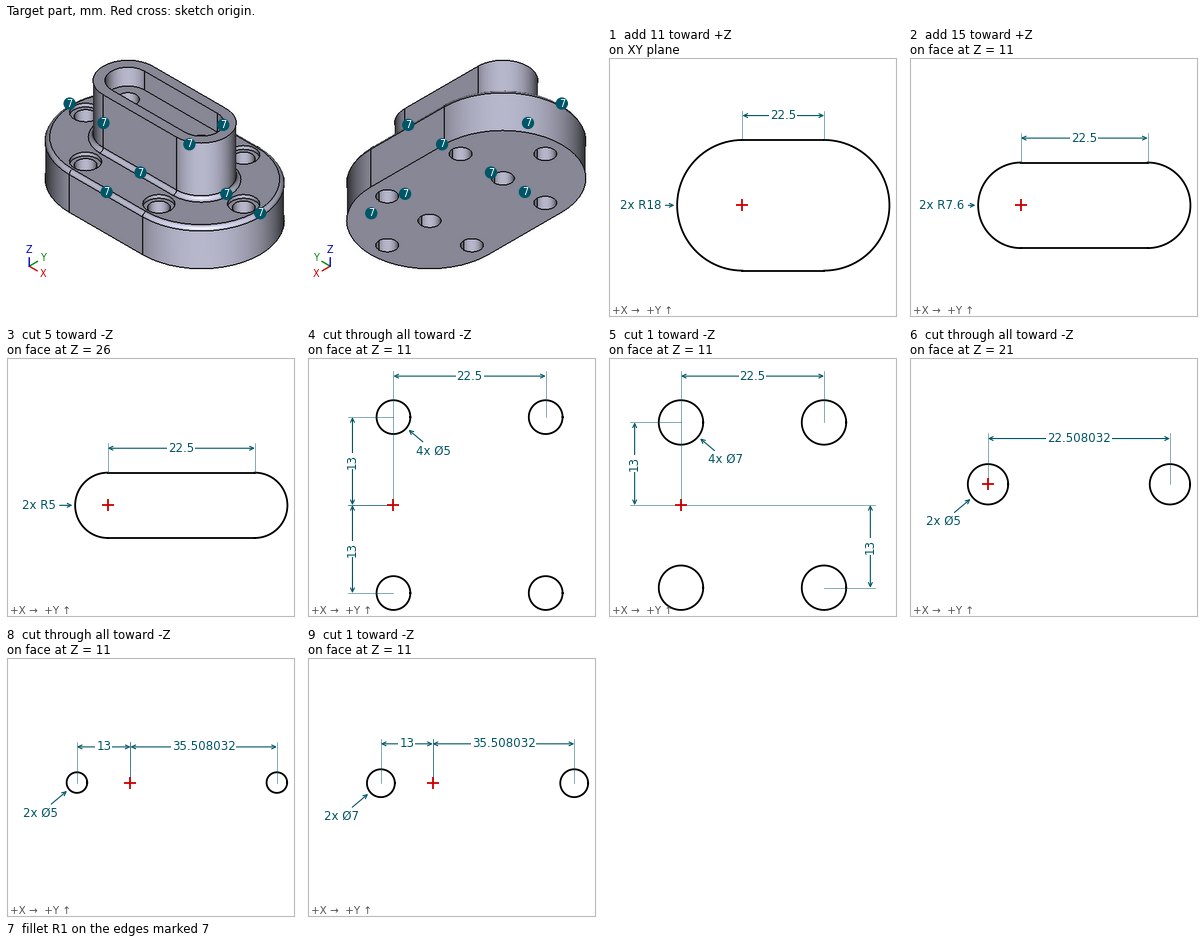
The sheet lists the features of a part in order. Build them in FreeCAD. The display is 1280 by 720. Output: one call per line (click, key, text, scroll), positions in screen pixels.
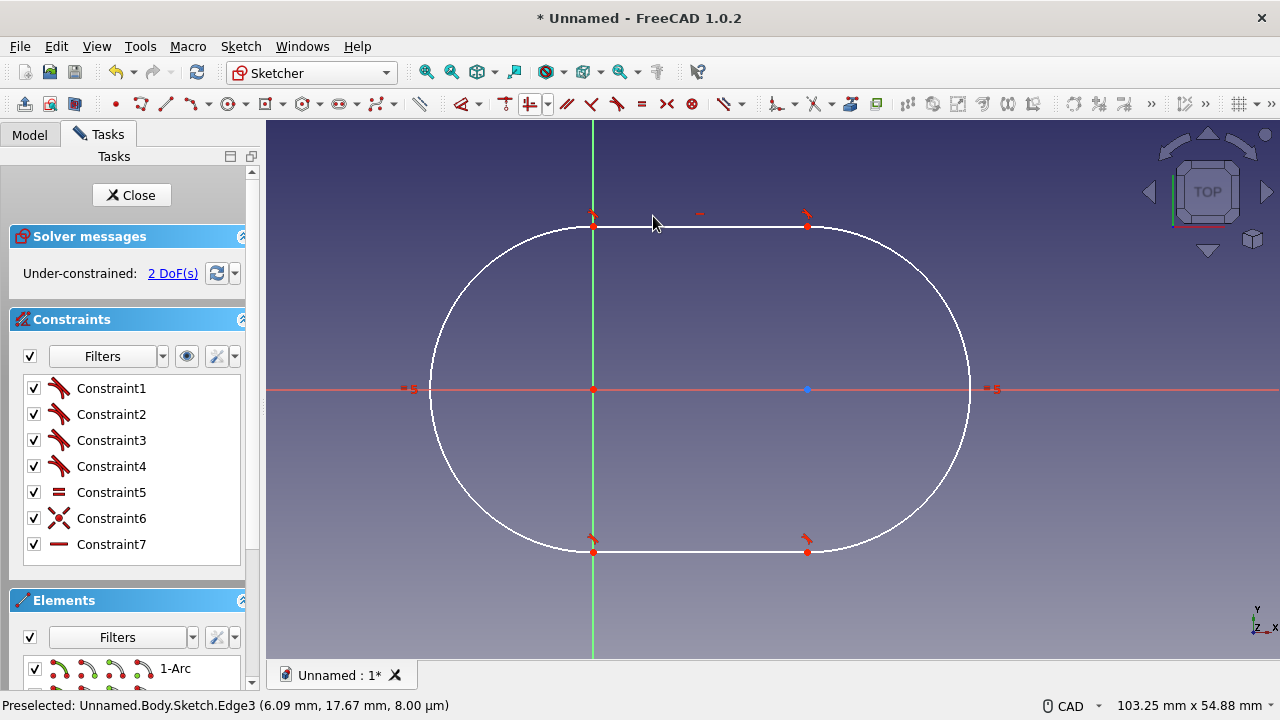
click(461, 294)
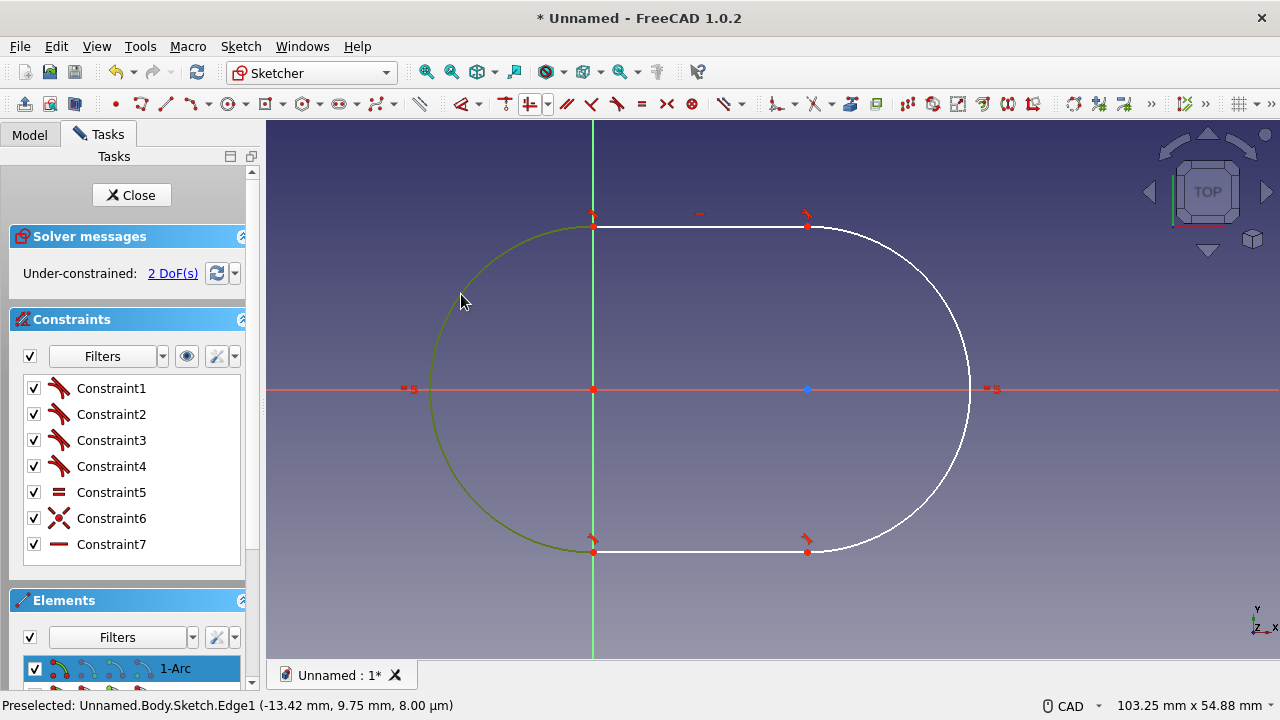
click(478, 104)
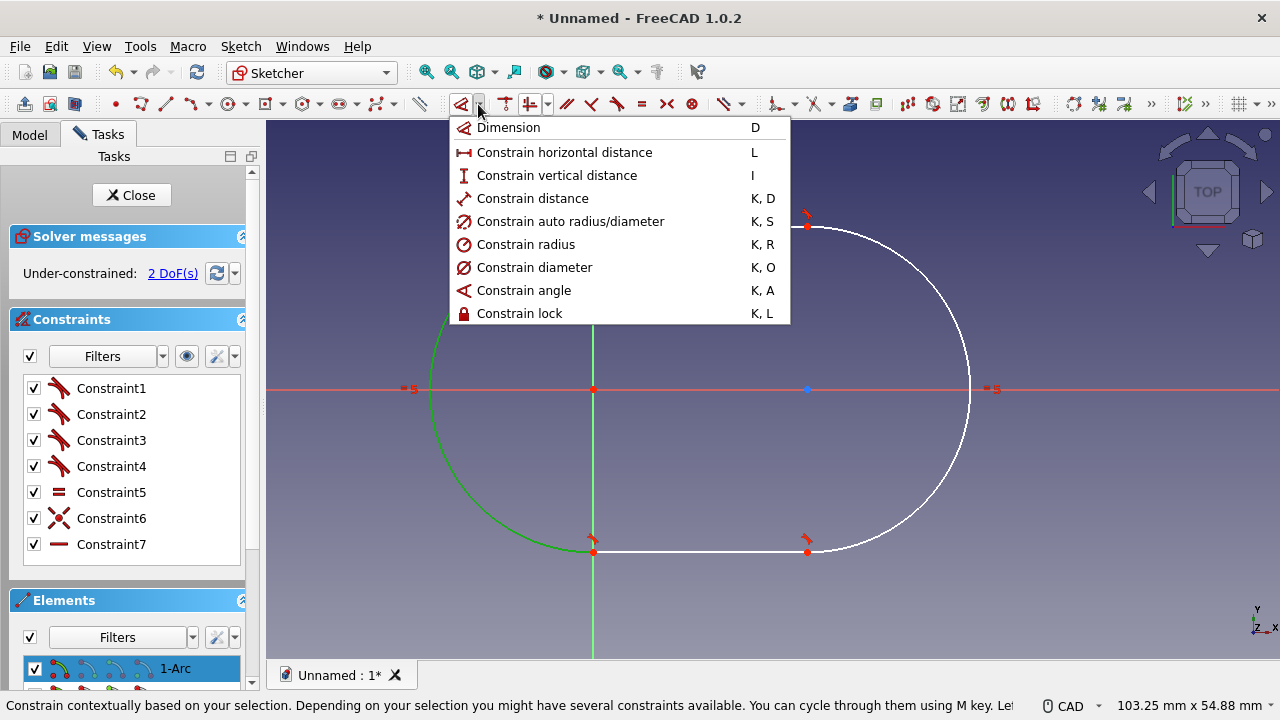
click(620, 244)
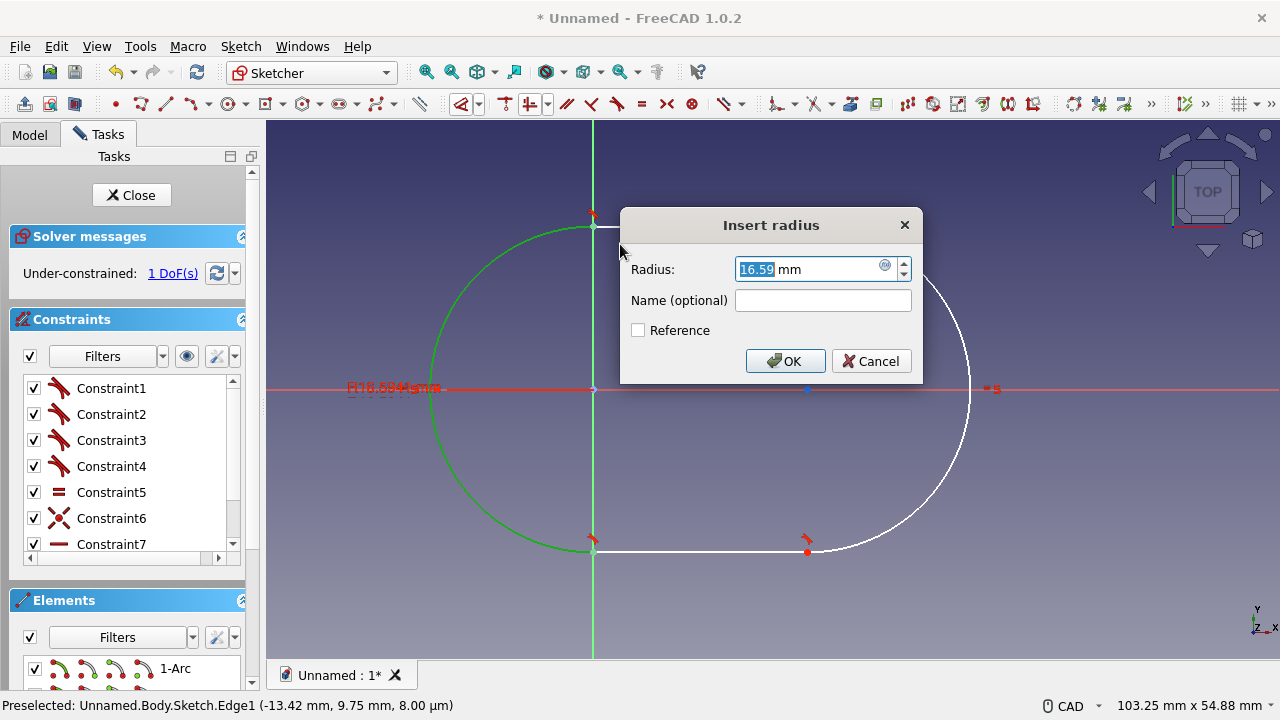
text(18)
key(Return)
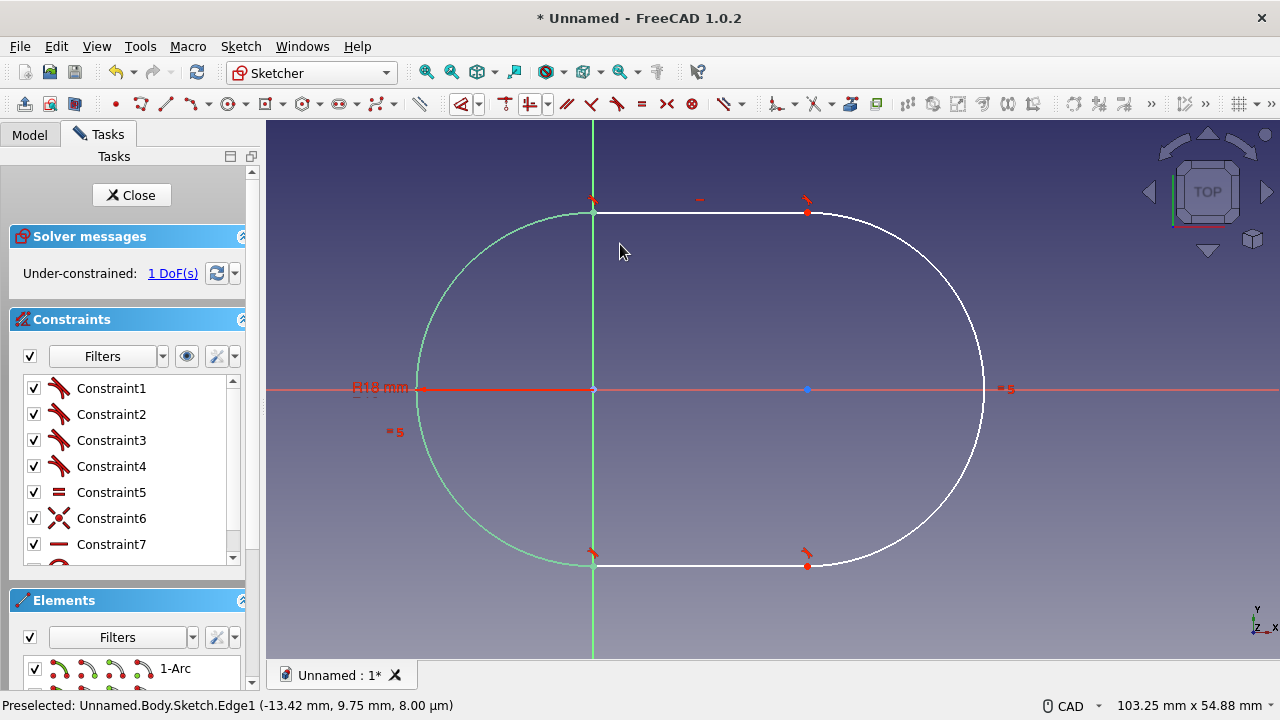
click(657, 213)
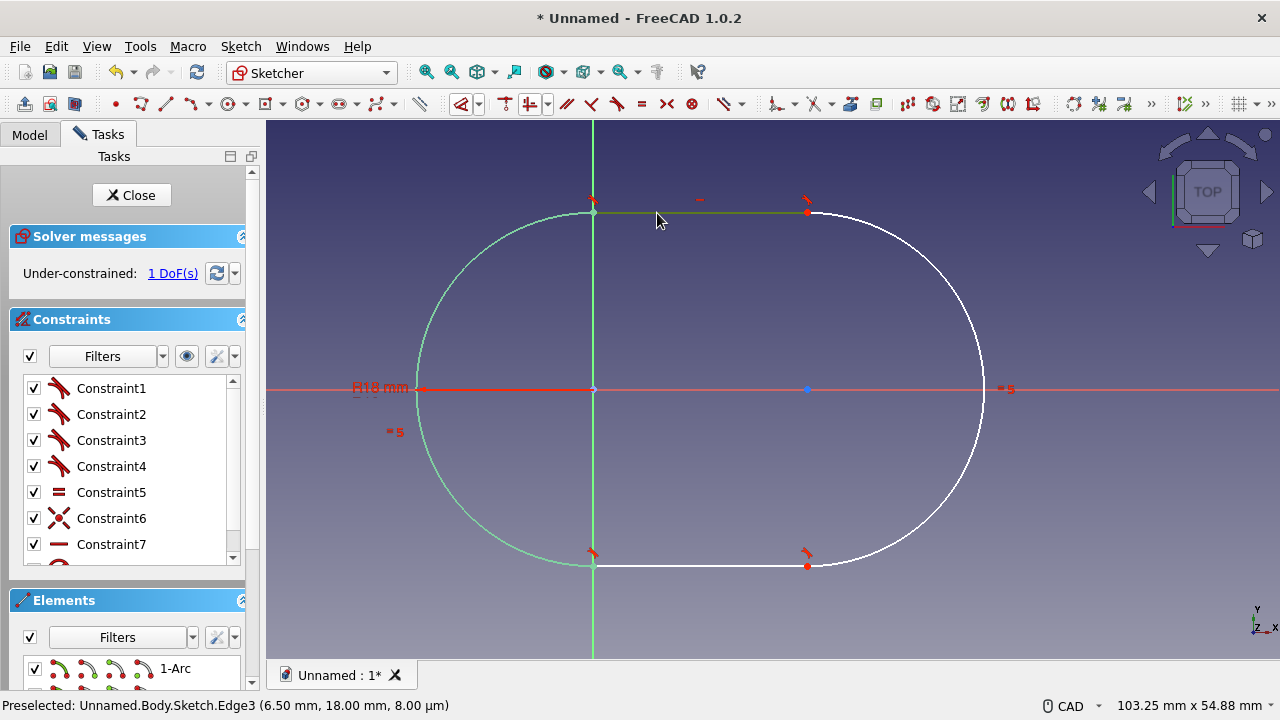
click(478, 104)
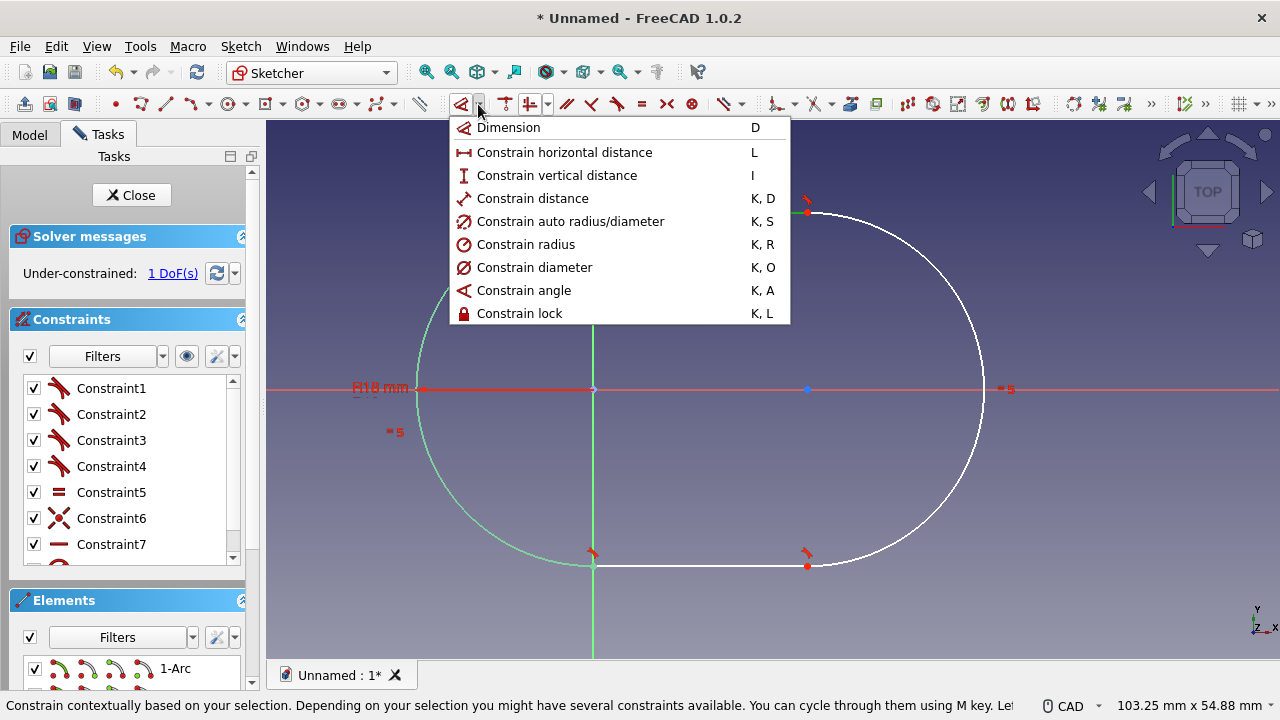
click(620, 152)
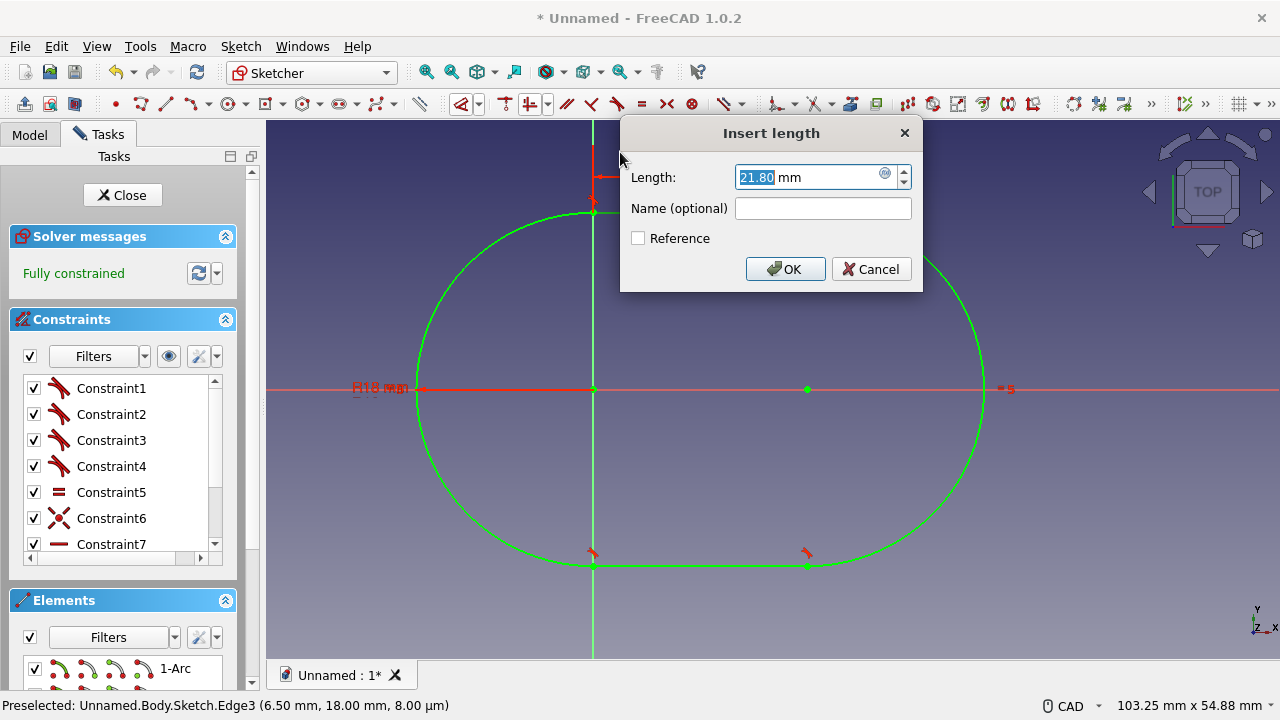
text(22.5)
key(Return)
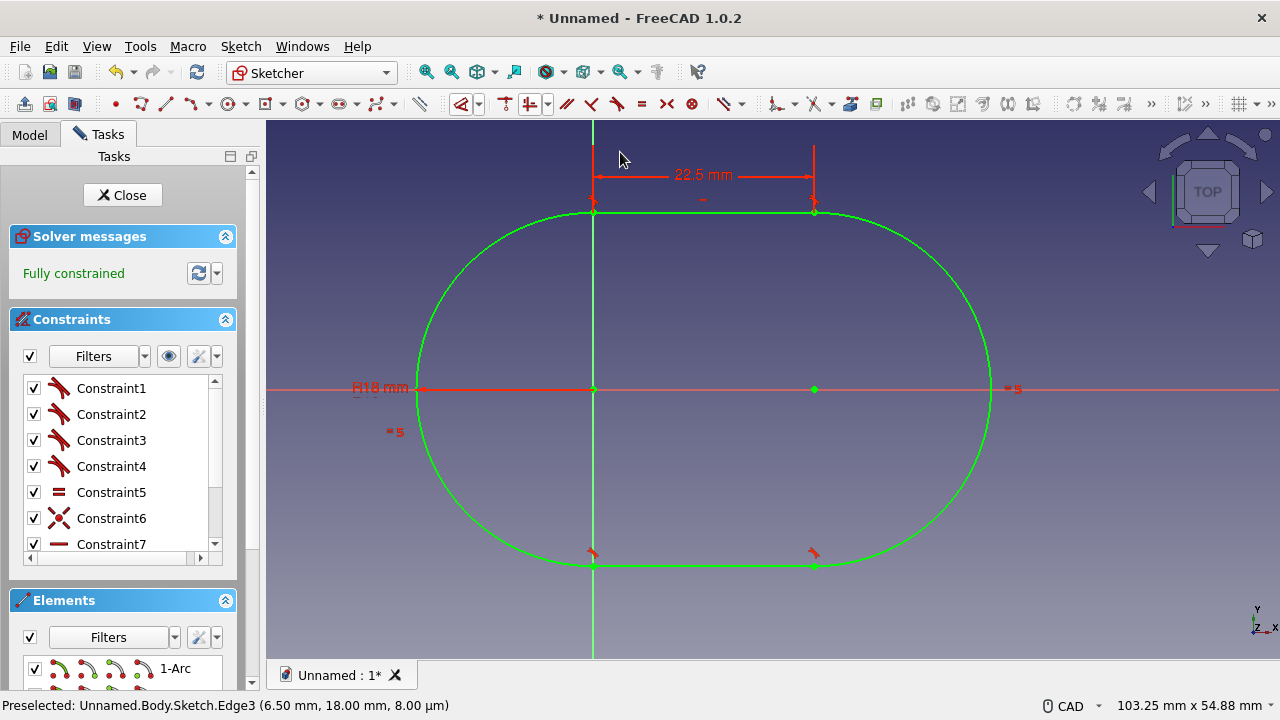
click(123, 195)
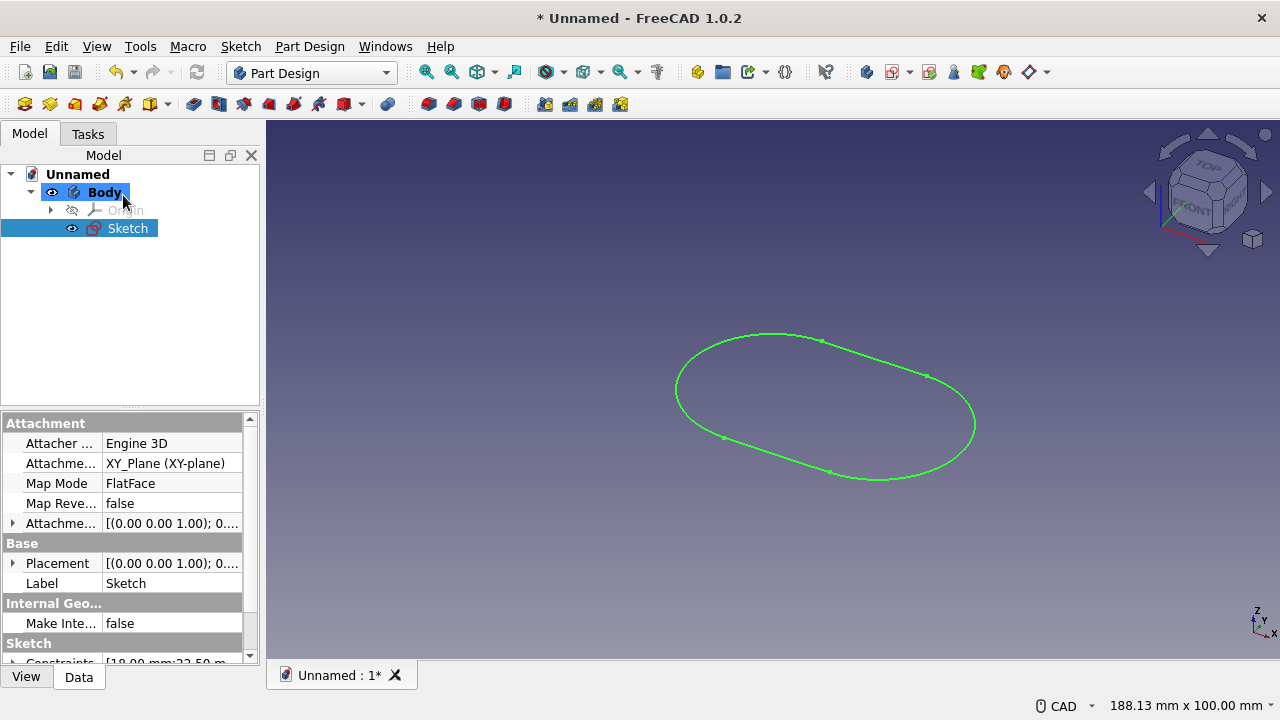
click(25, 104)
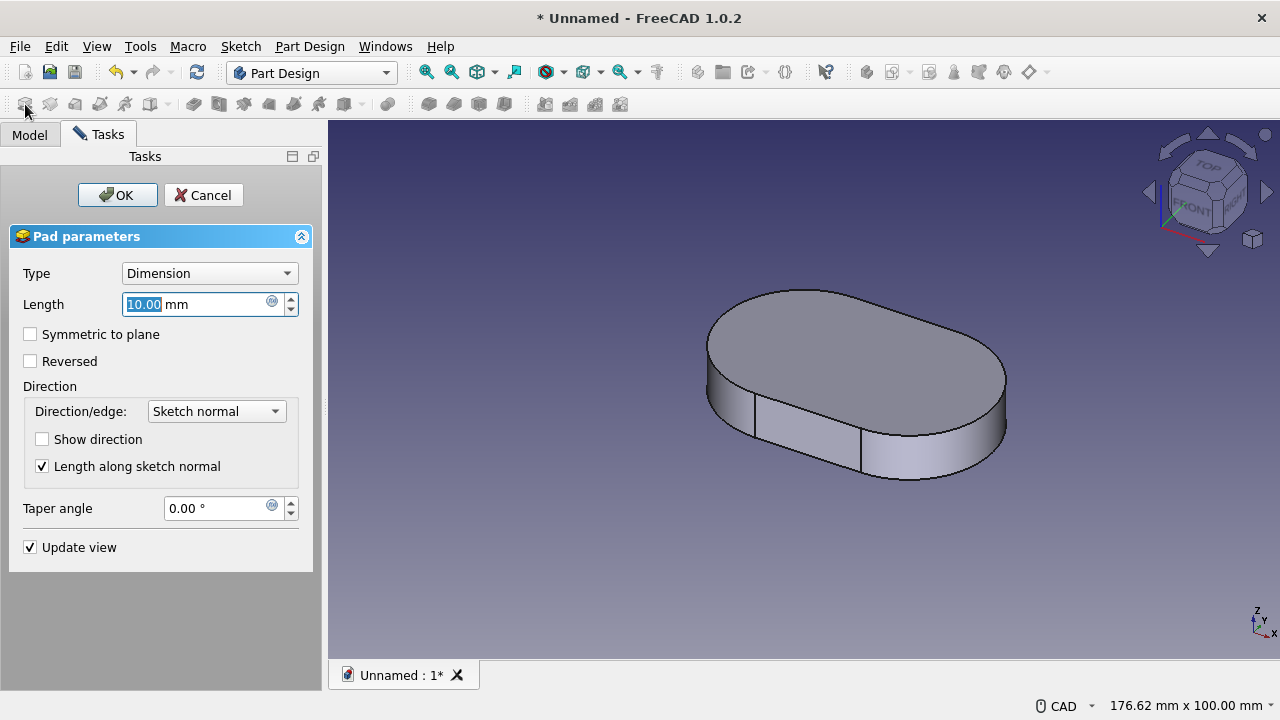
text(11)
key(Tab)